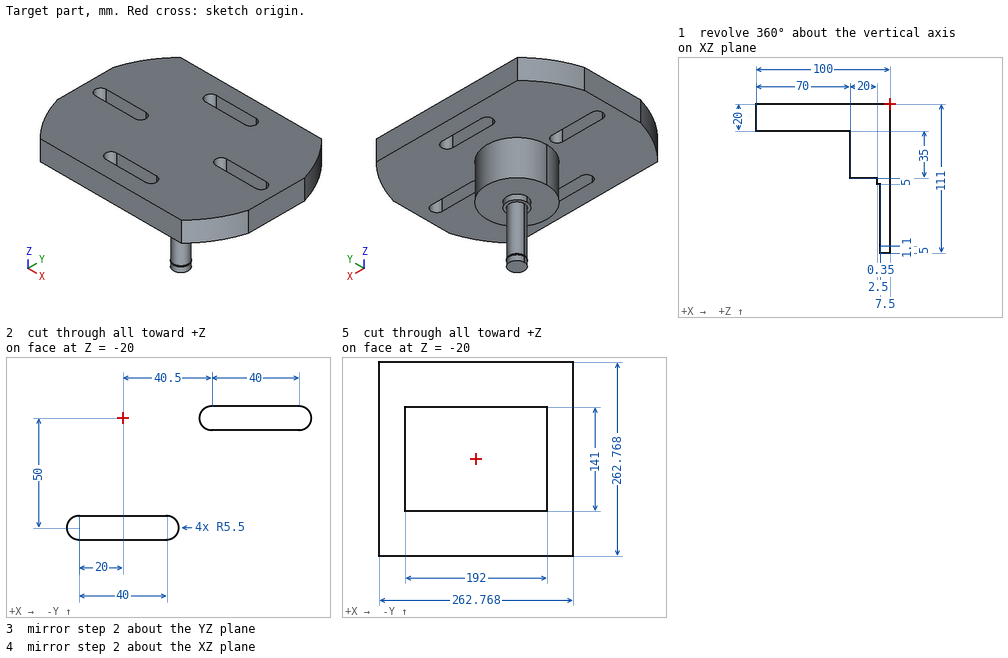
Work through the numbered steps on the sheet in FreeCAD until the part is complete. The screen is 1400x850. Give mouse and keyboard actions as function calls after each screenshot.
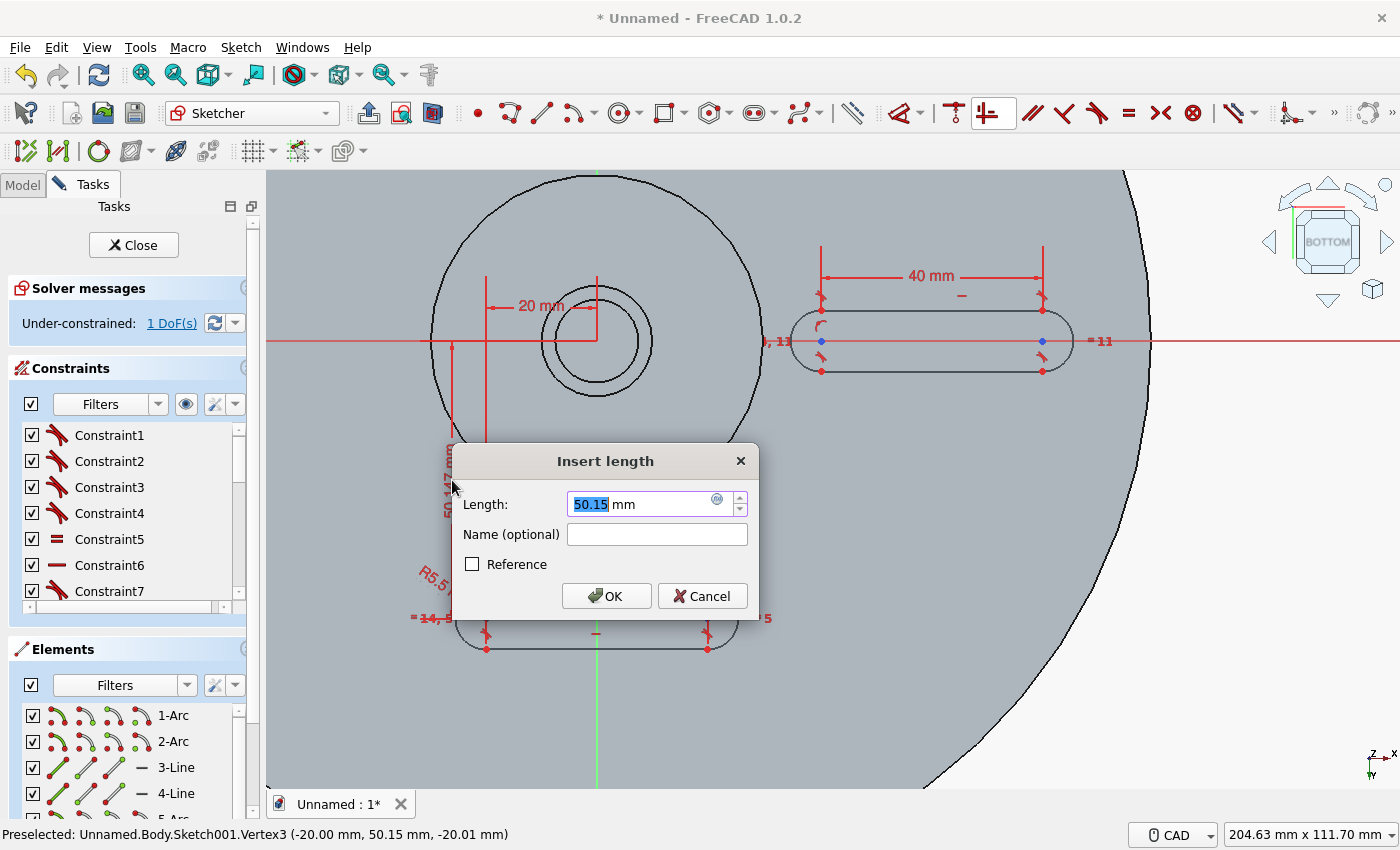
text(50)
key(Return)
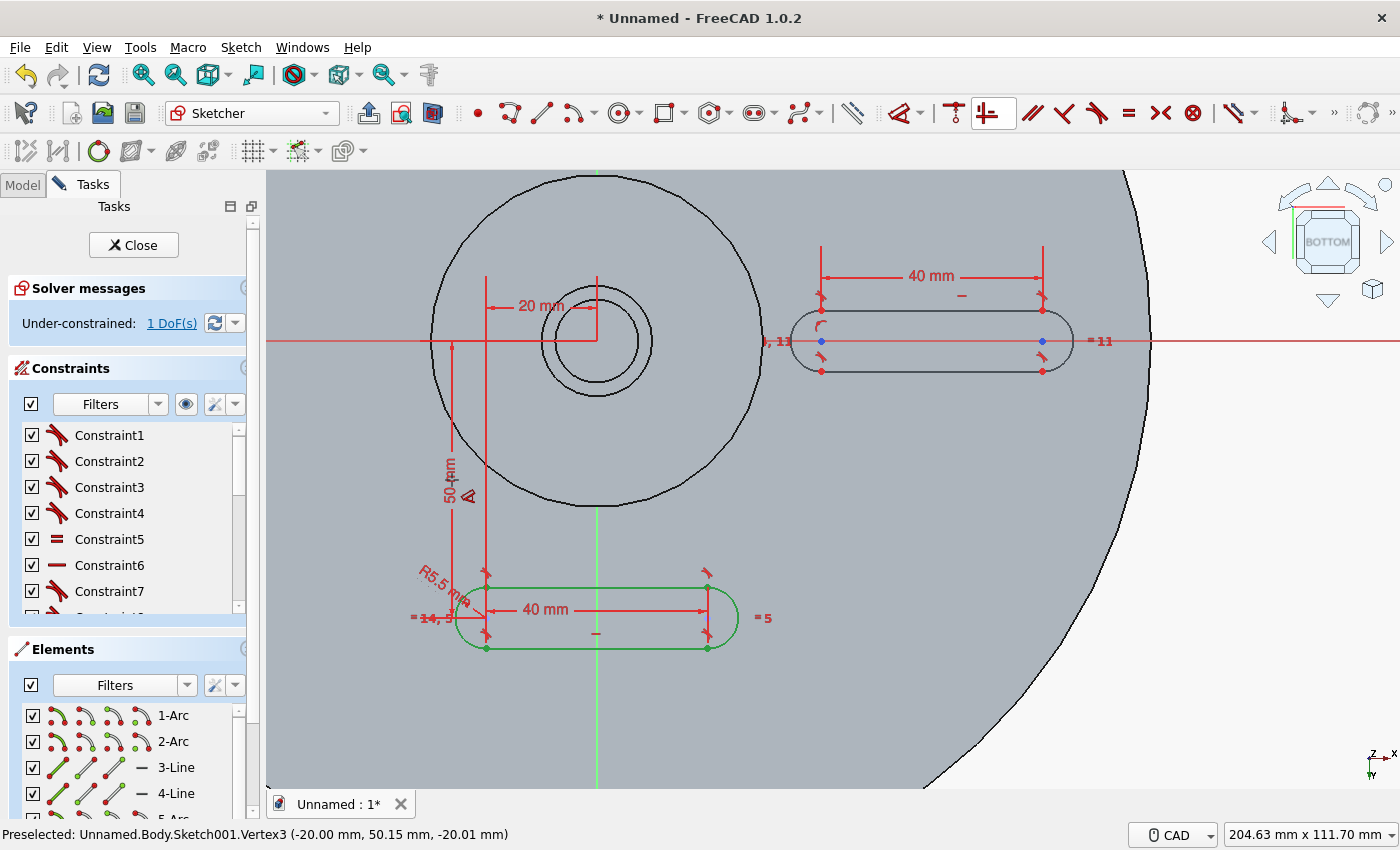
click(821, 311)
click(709, 277)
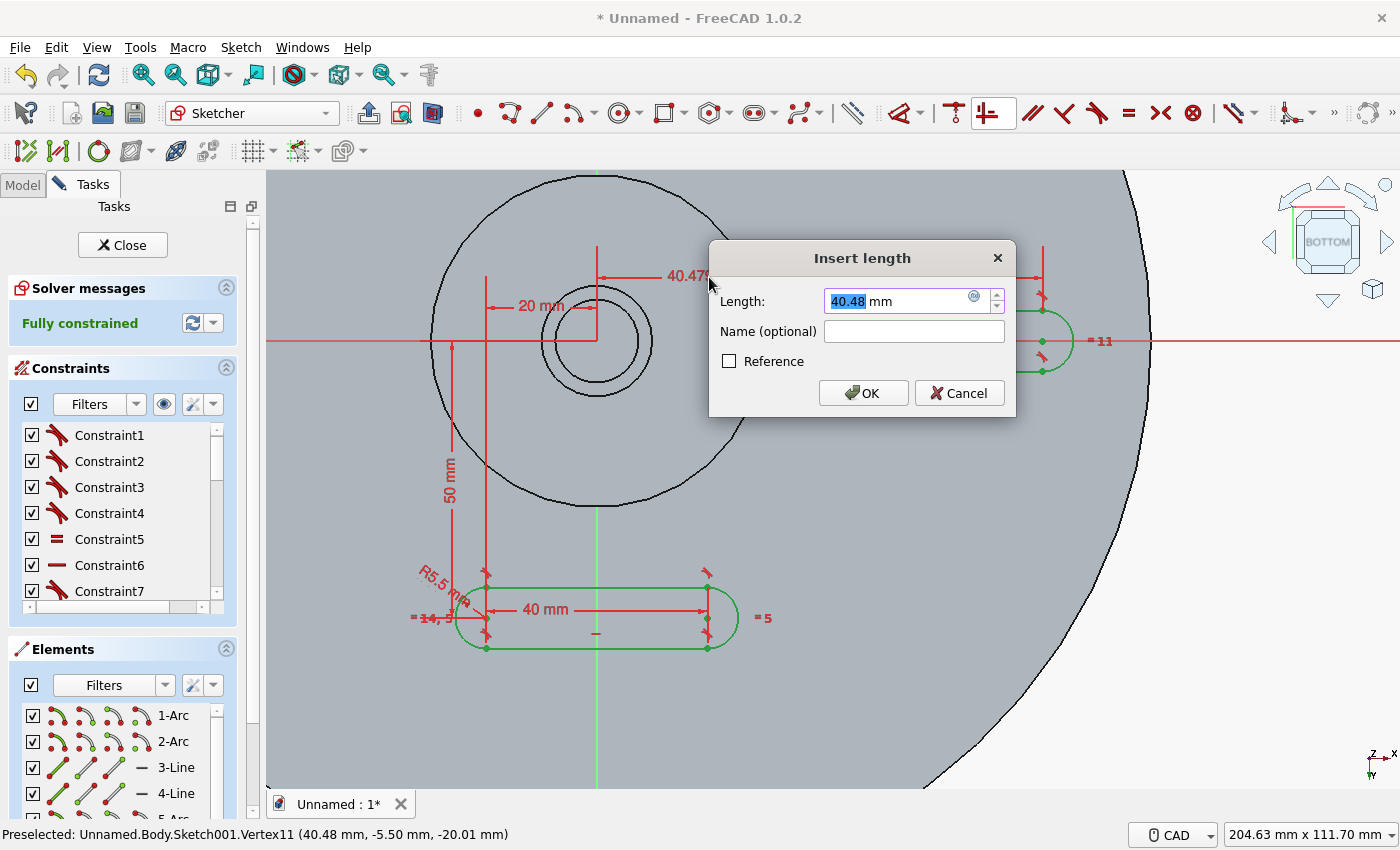
text(40.5)
key(Return)
key(Escape)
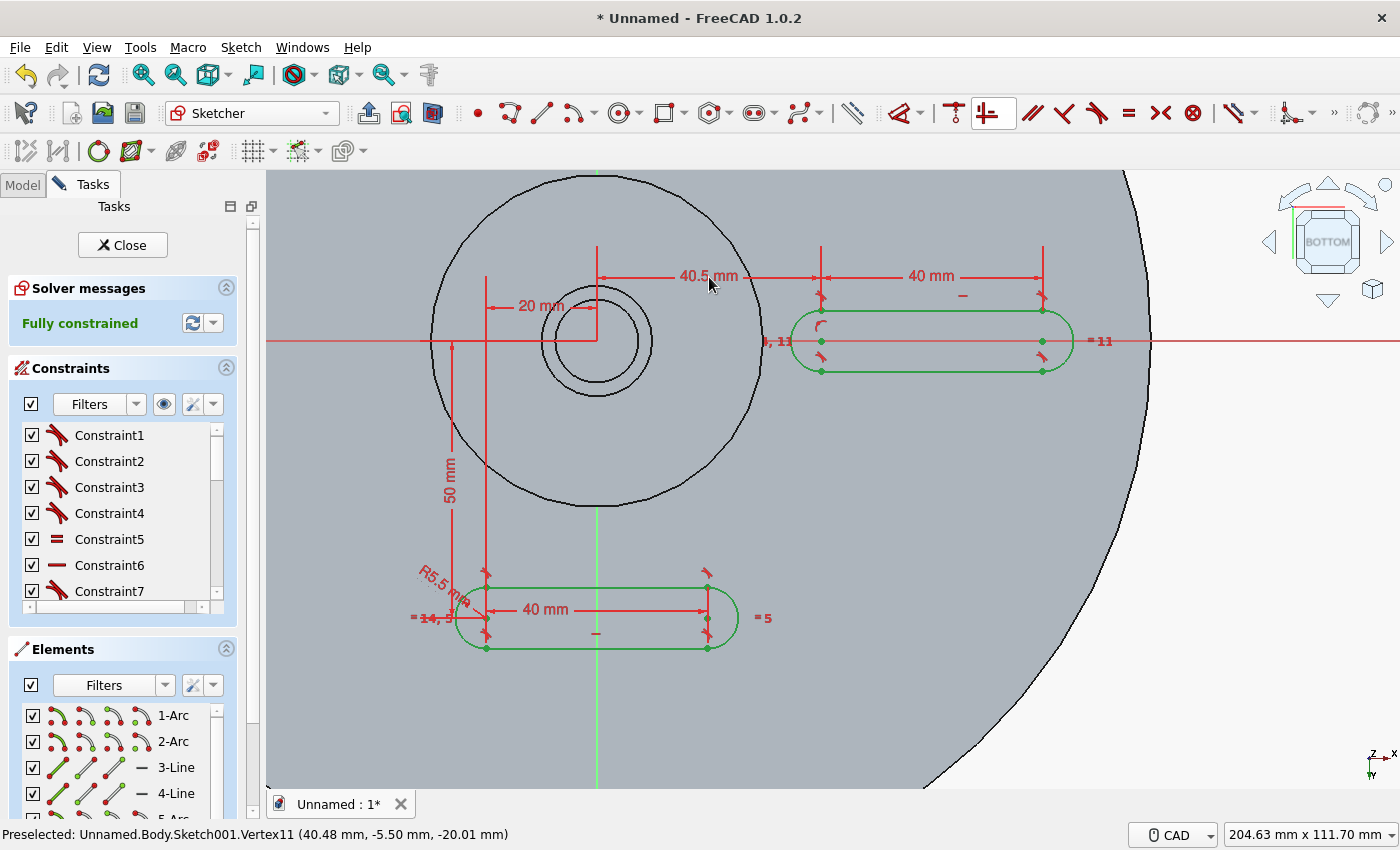
click(123, 245)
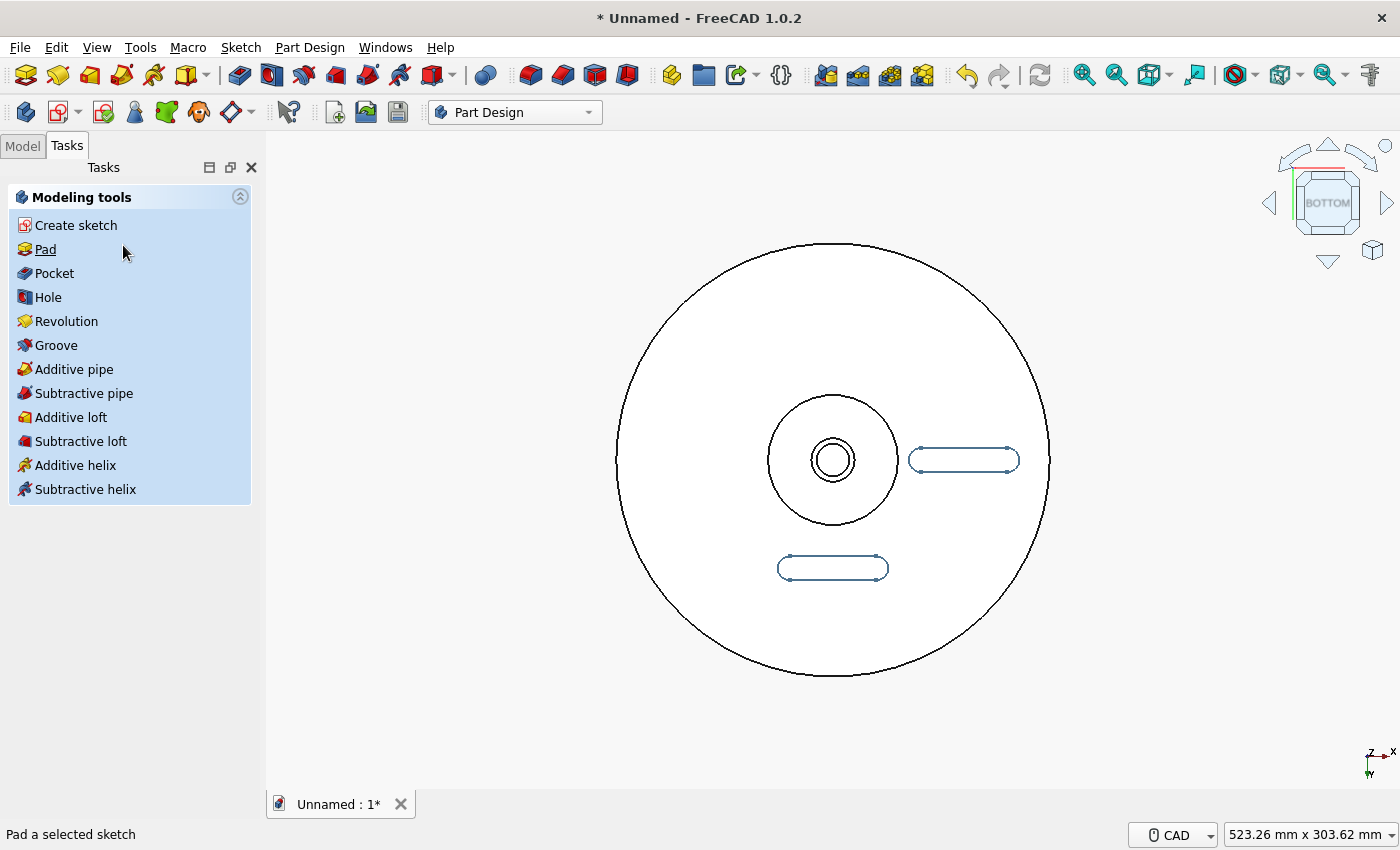
click(240, 76)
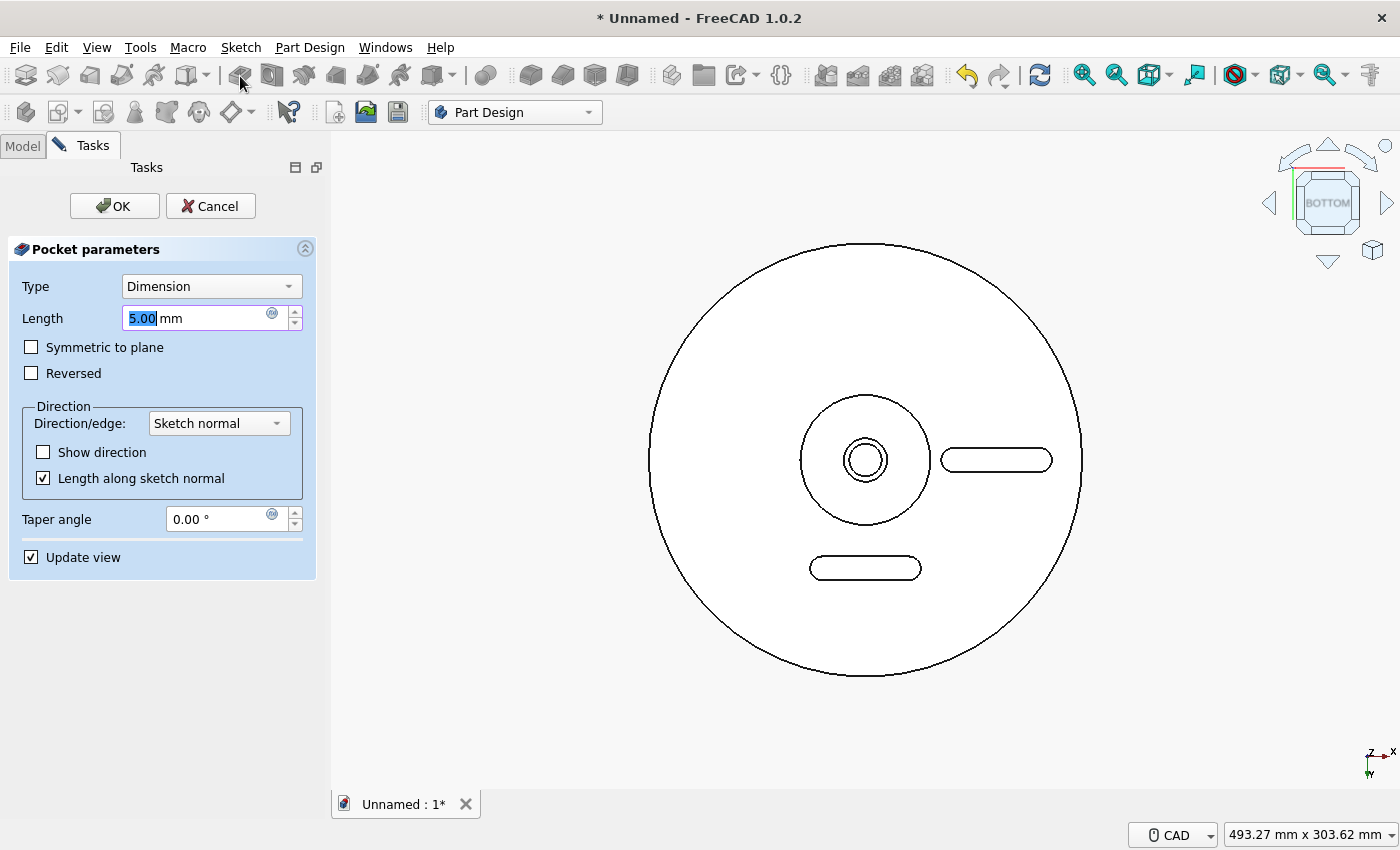
click(212, 286)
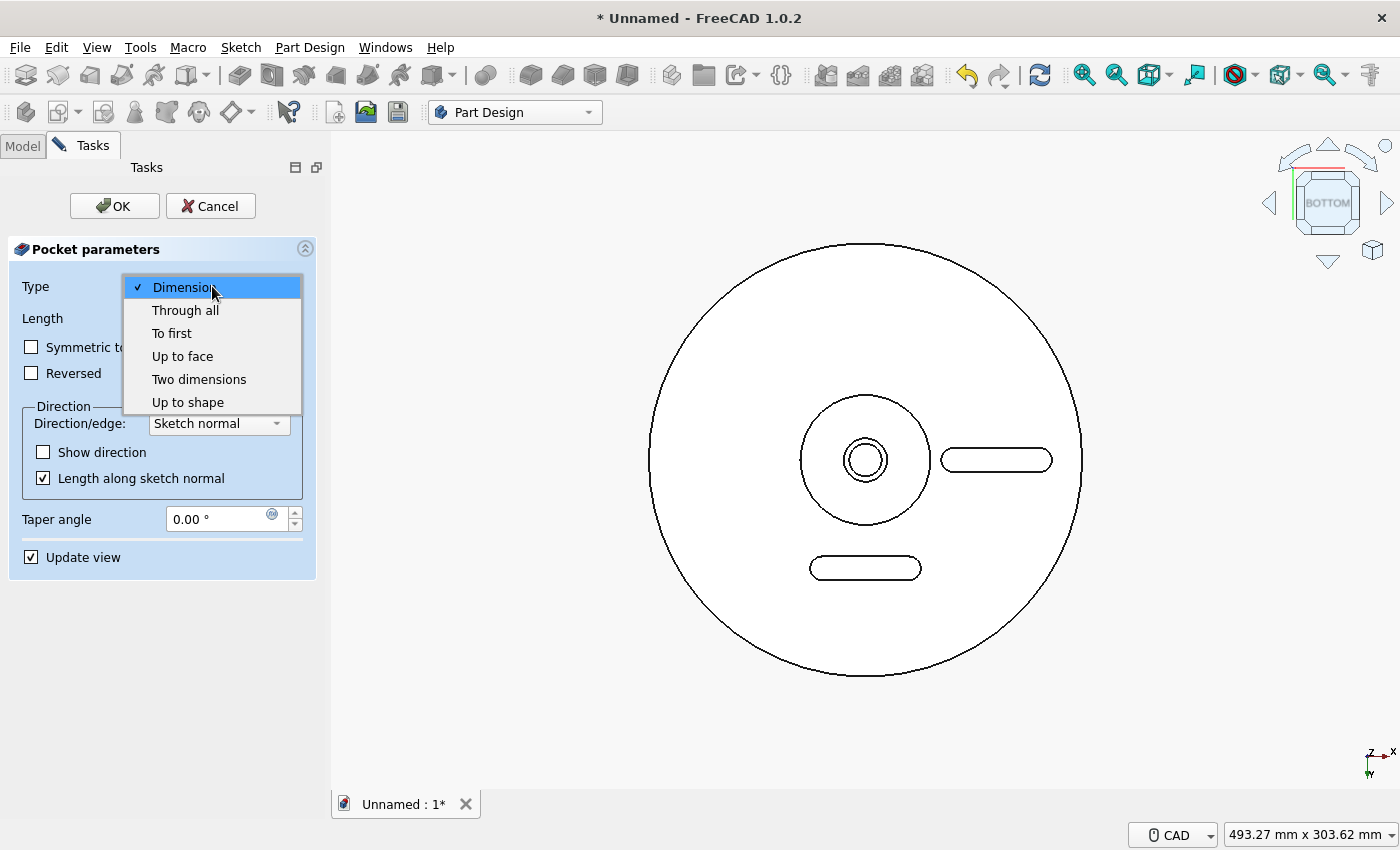
click(212, 310)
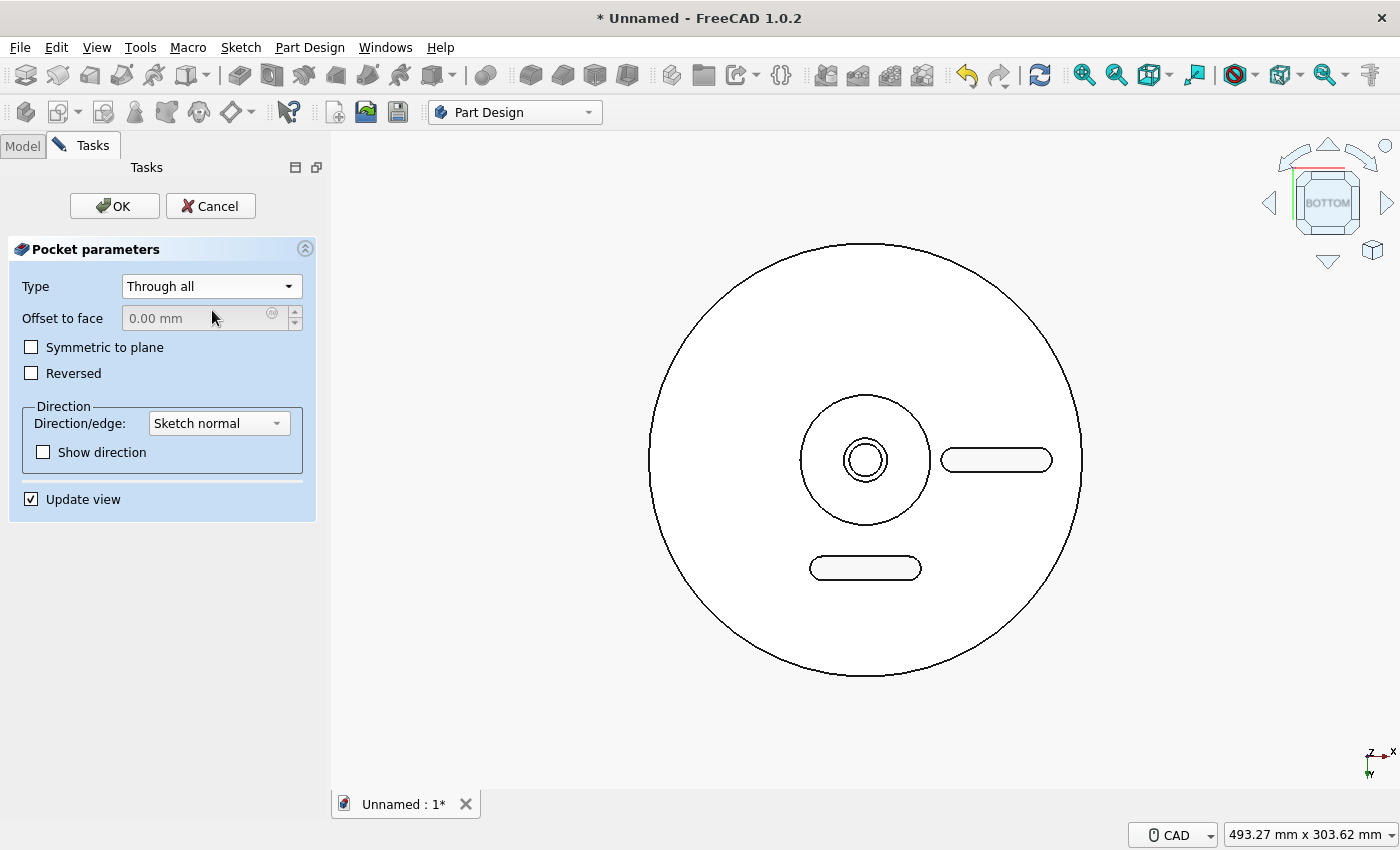
click(115, 206)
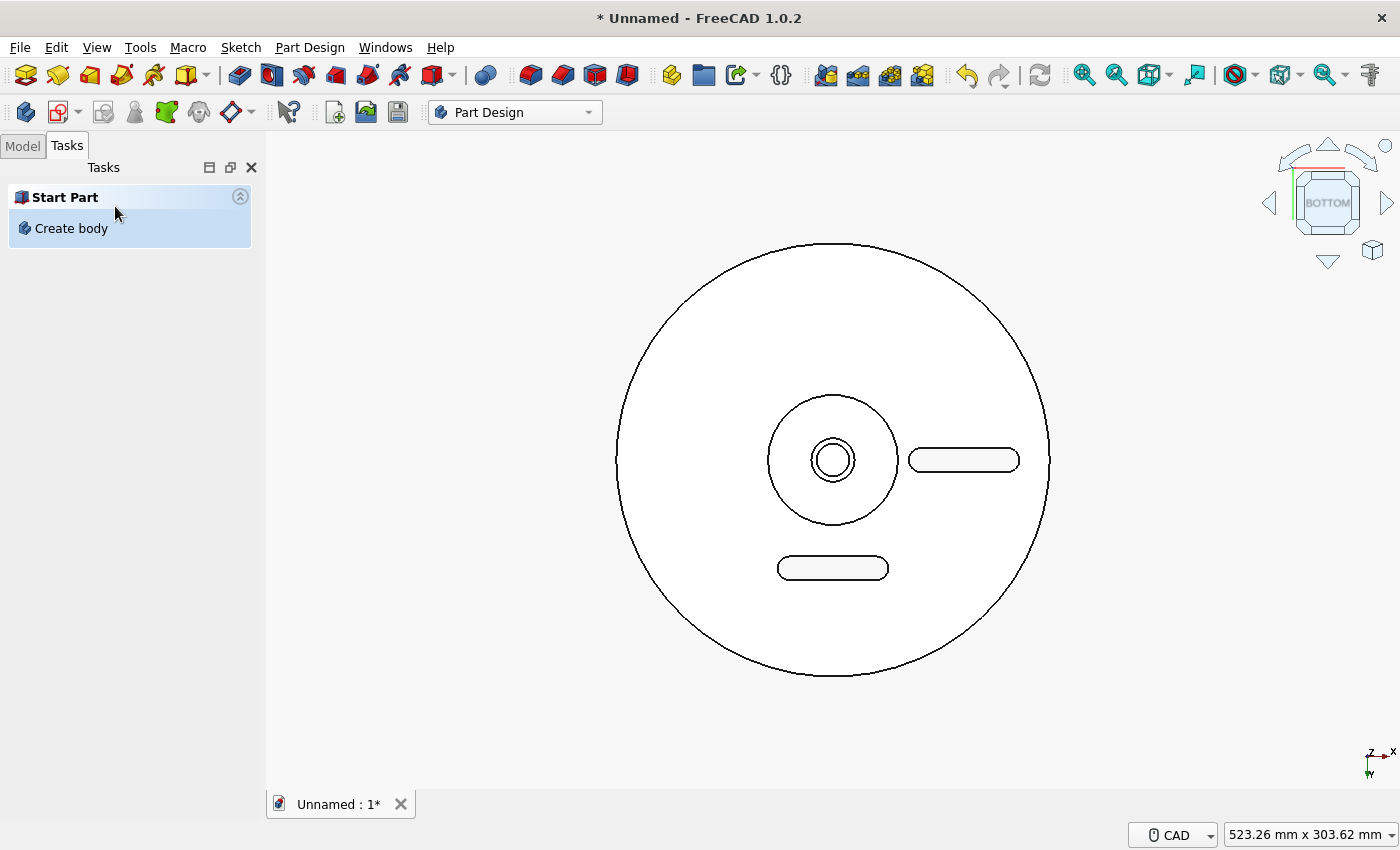
click(23, 145)